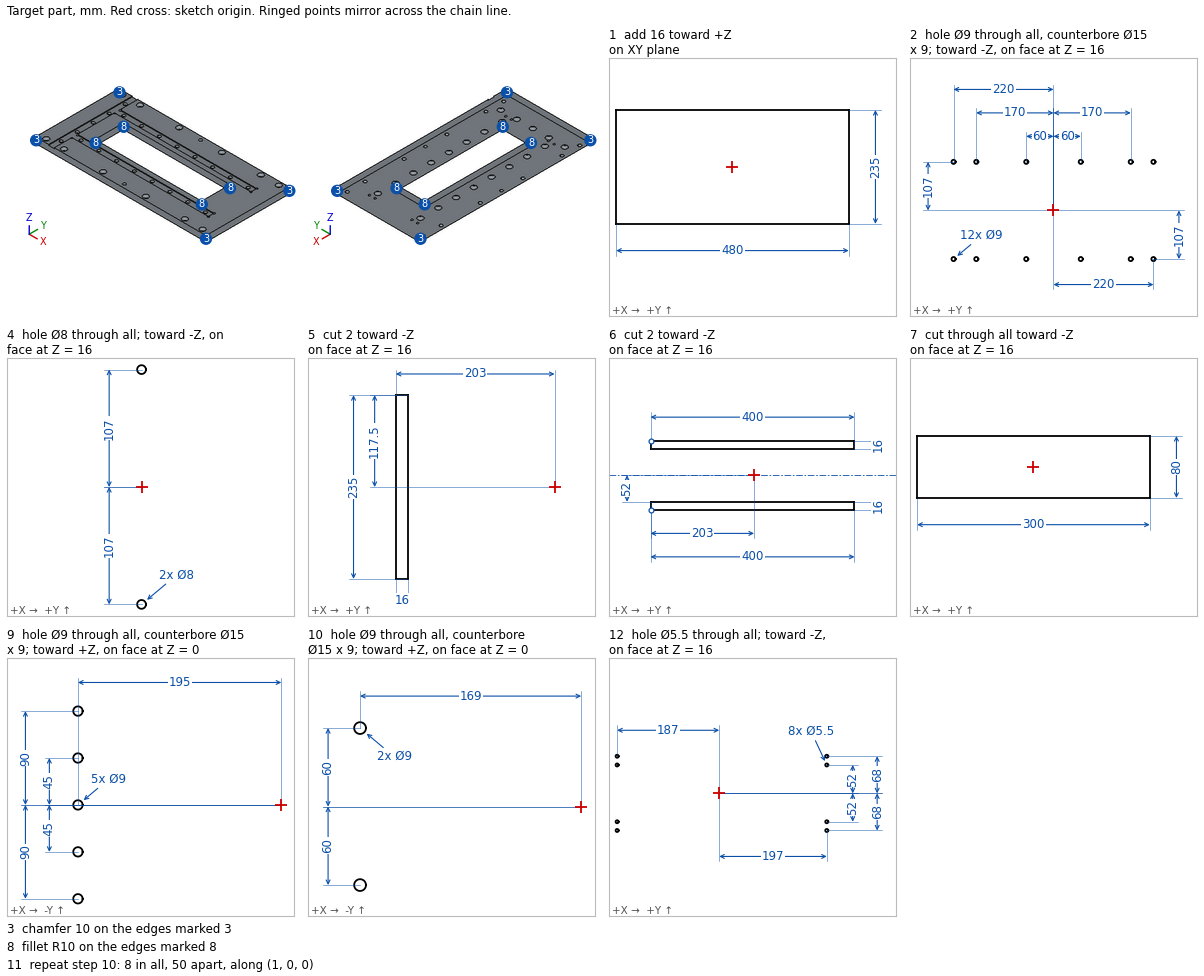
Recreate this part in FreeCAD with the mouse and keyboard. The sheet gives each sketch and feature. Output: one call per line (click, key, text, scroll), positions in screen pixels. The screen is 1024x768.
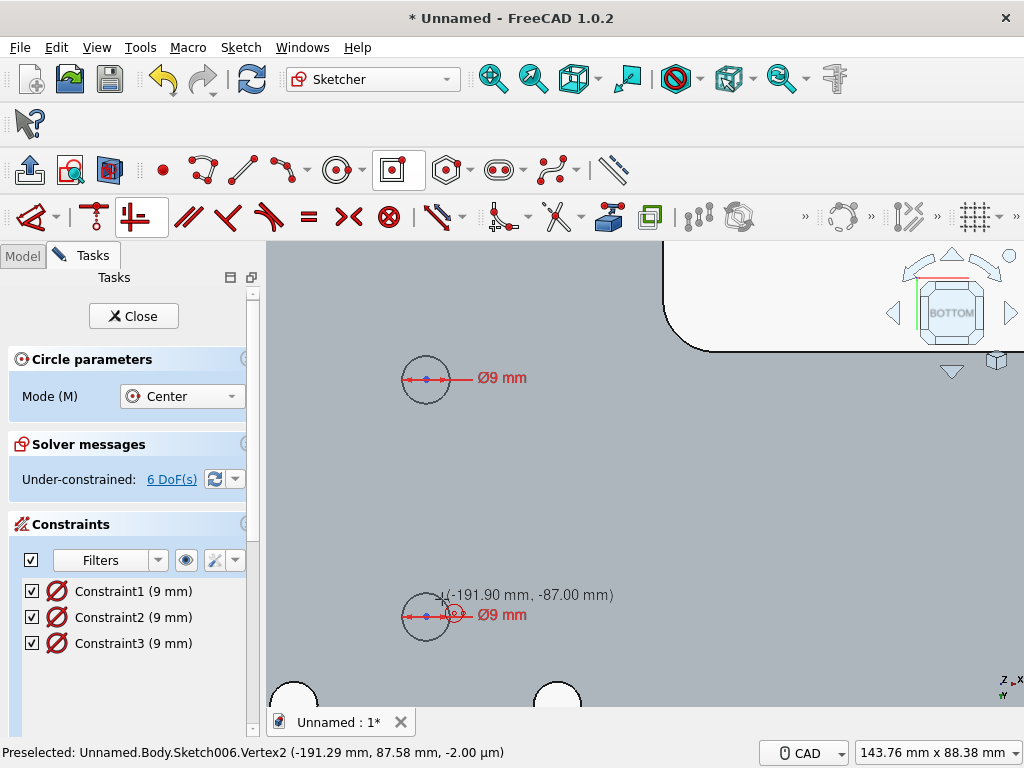
scroll(425, 617, down, 6)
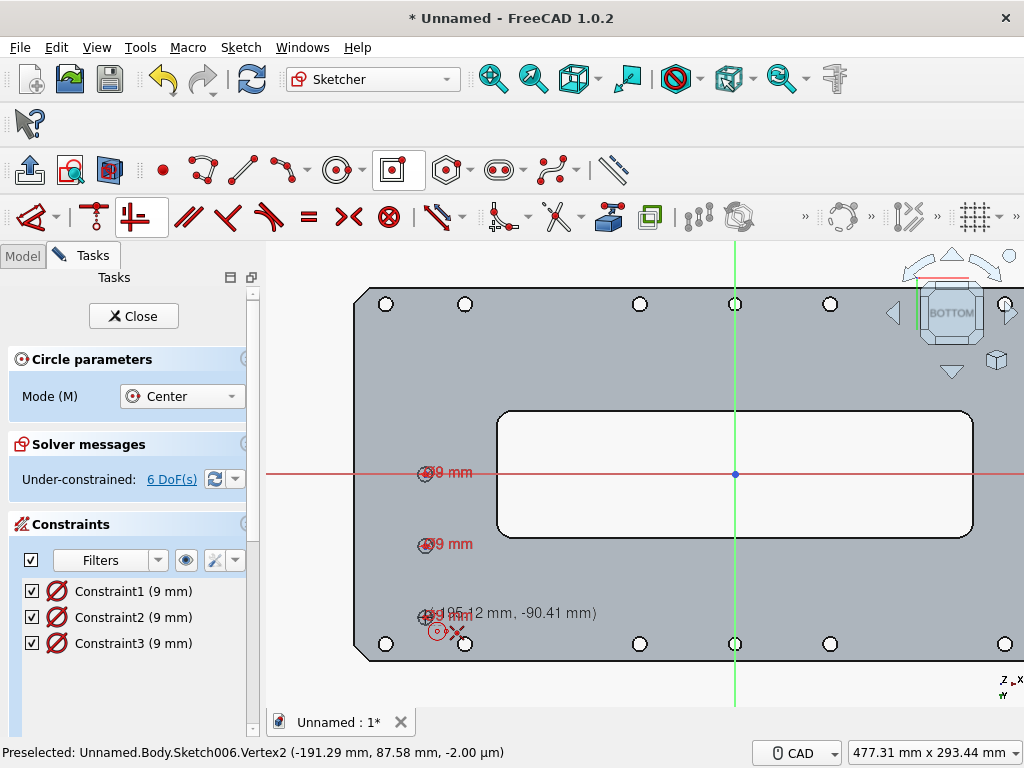
scroll(425, 331, up, 6)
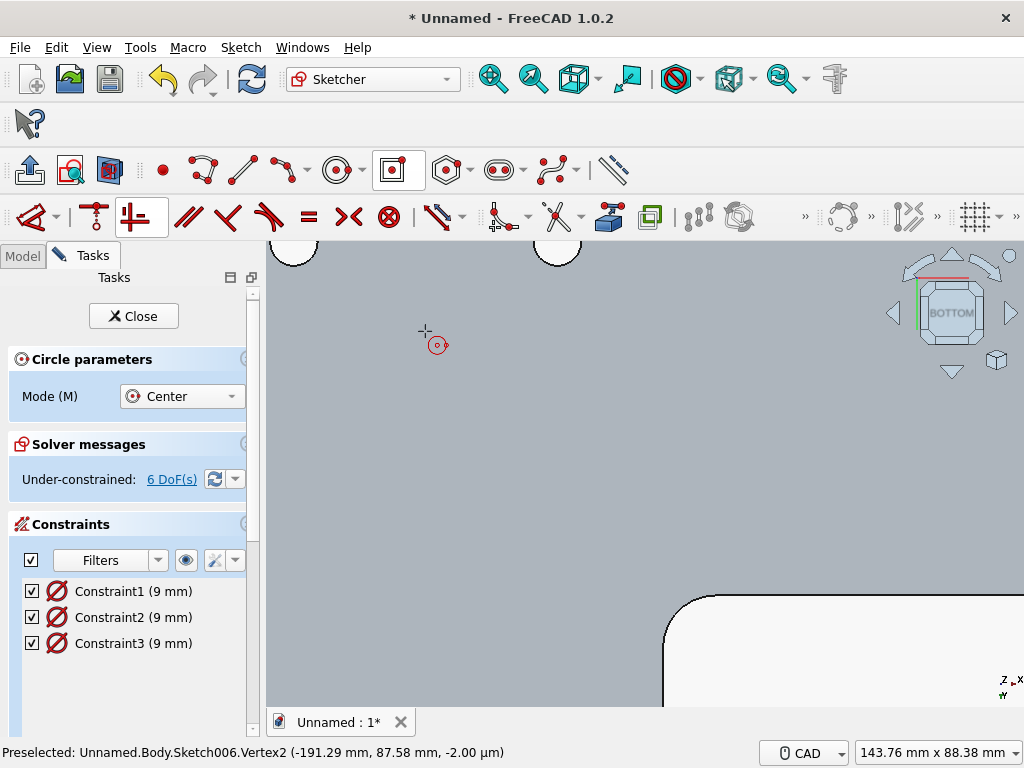
click(426, 332)
move(442, 315)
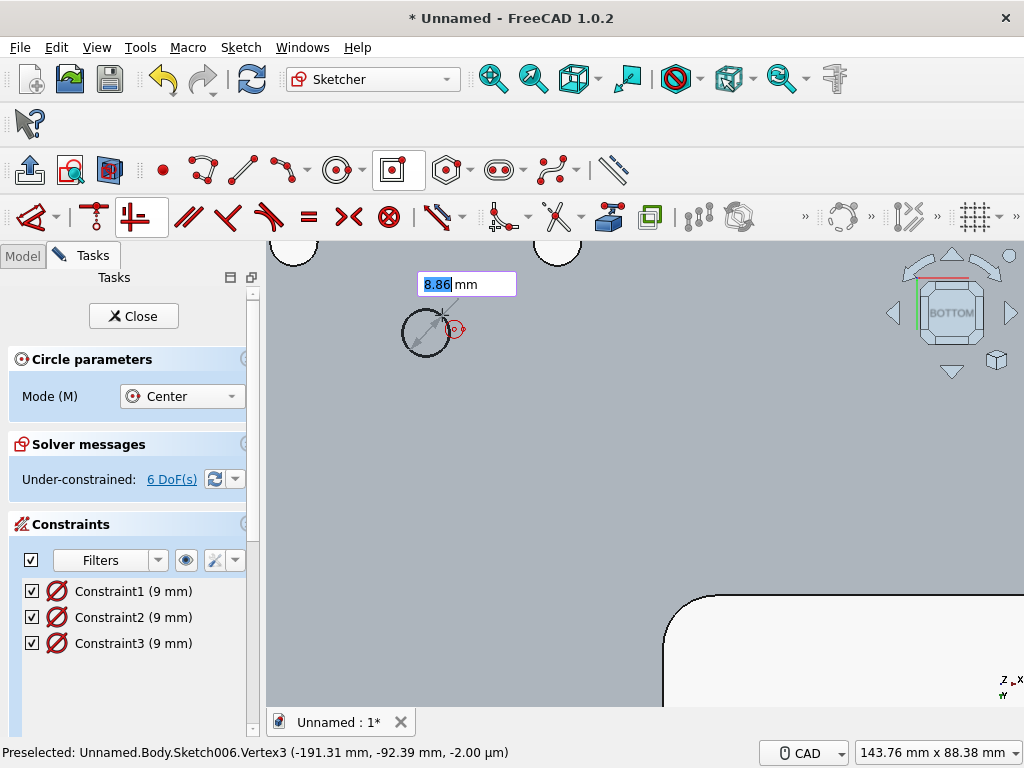
text(9)
key(Return)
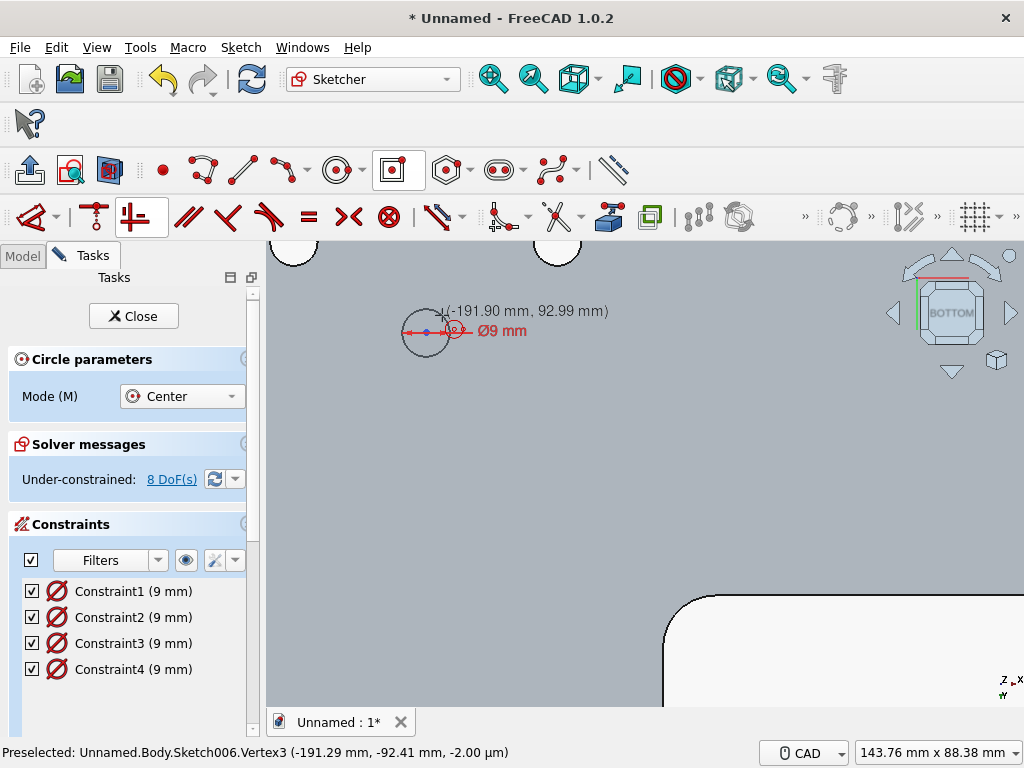
click(426, 569)
move(442, 552)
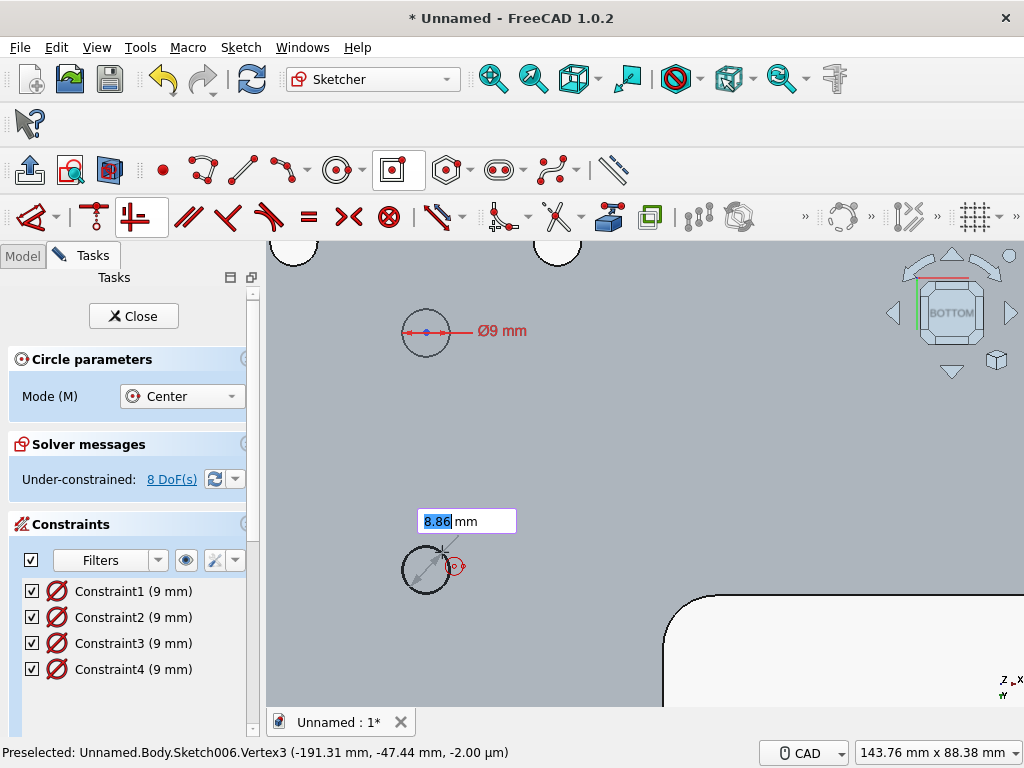
text(9)
key(Return)
key(Escape)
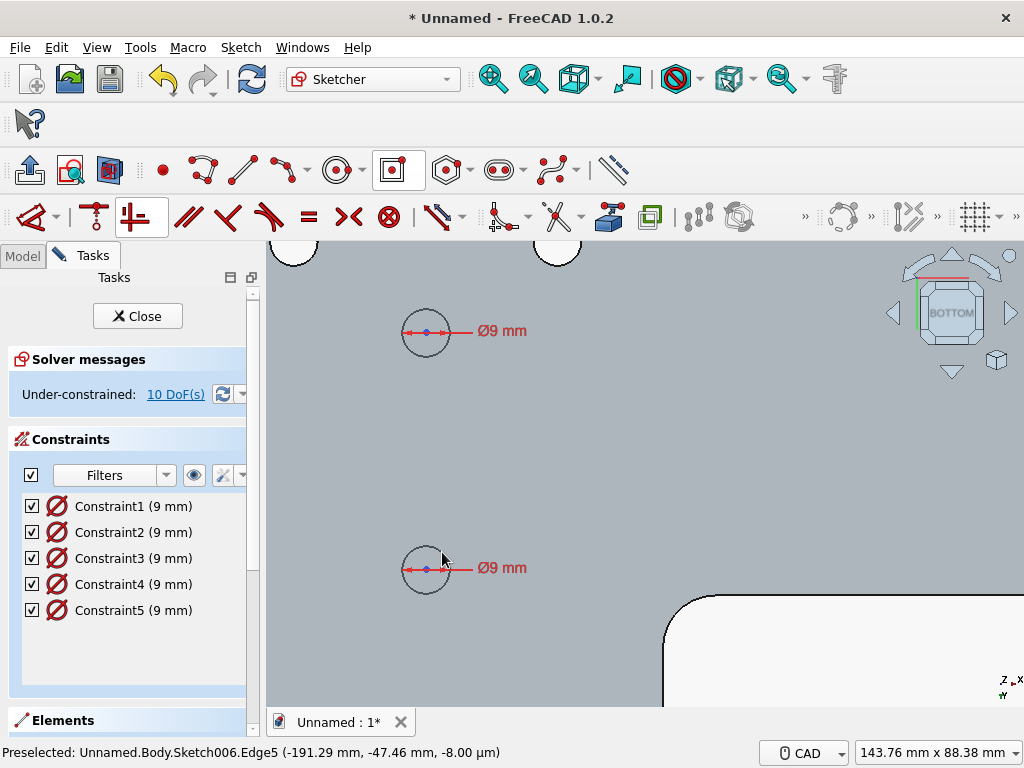
scroll(425, 331, down, 6)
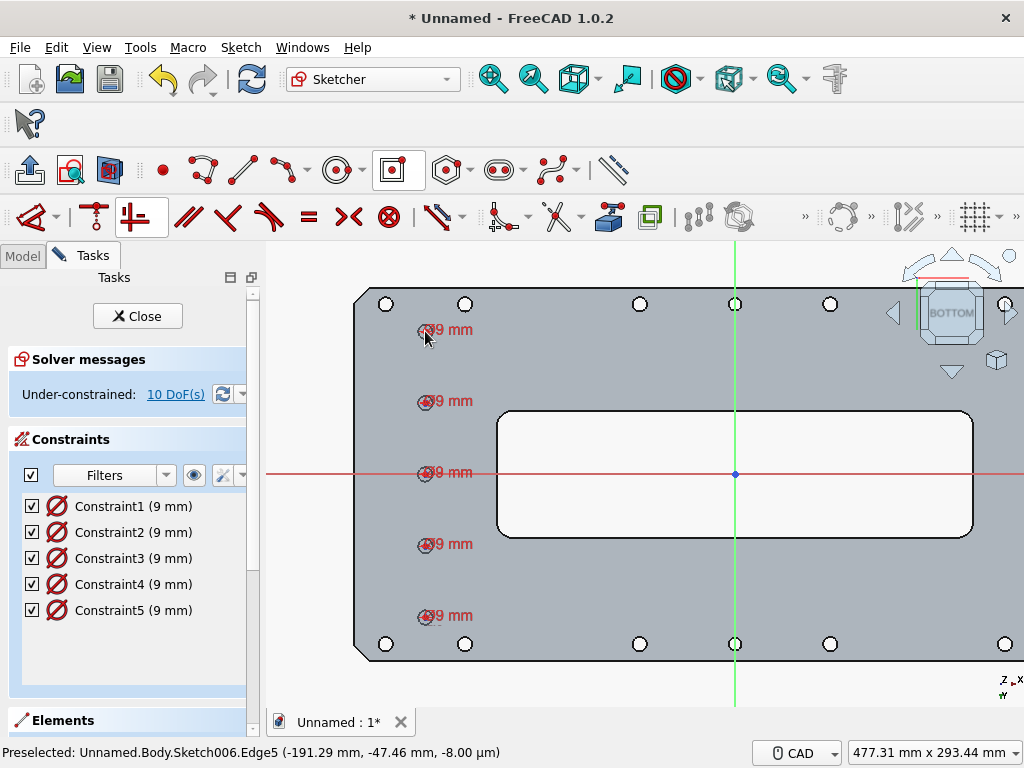
click(425, 474)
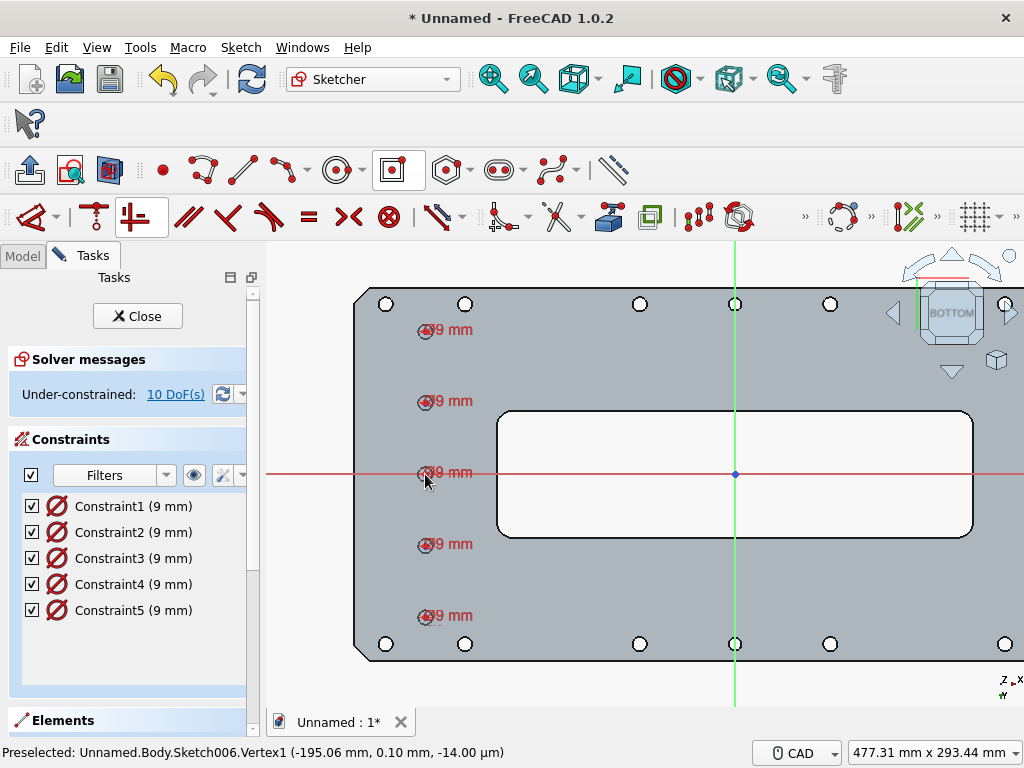
click(334, 474)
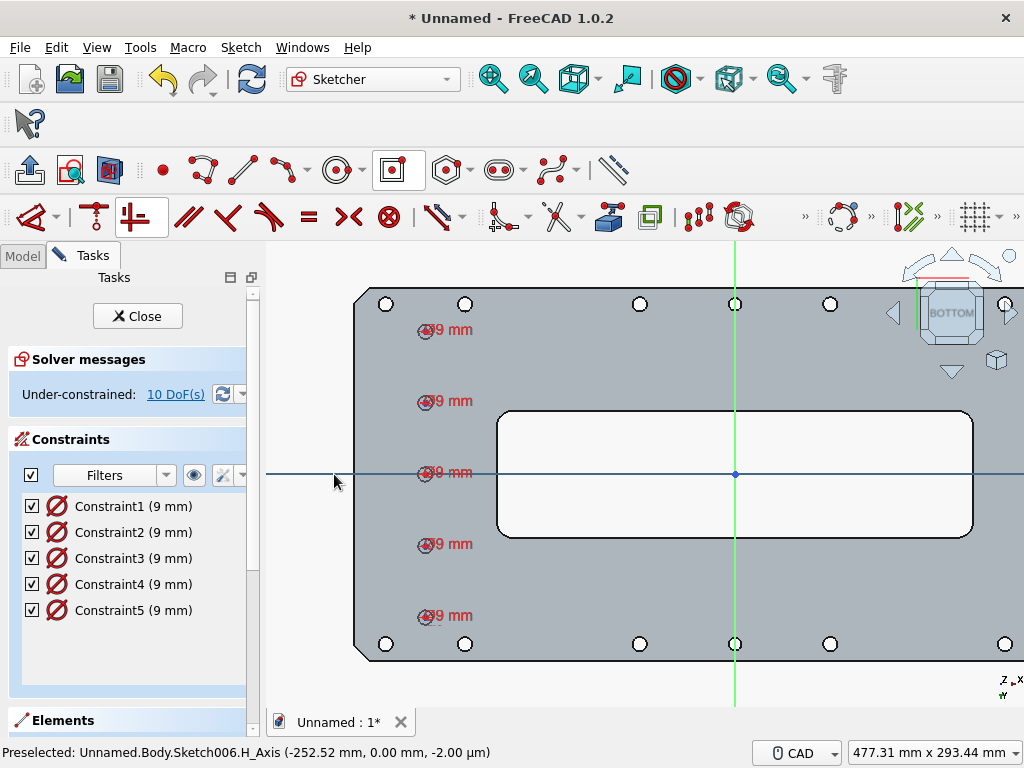
click(94, 218)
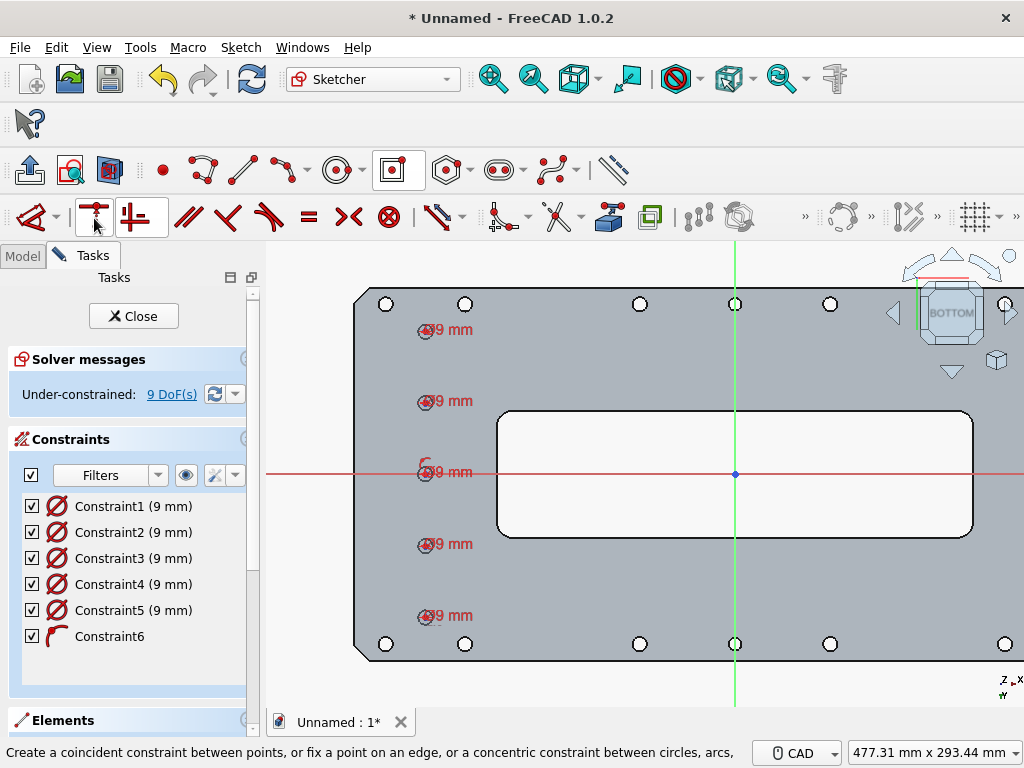
click(425, 474)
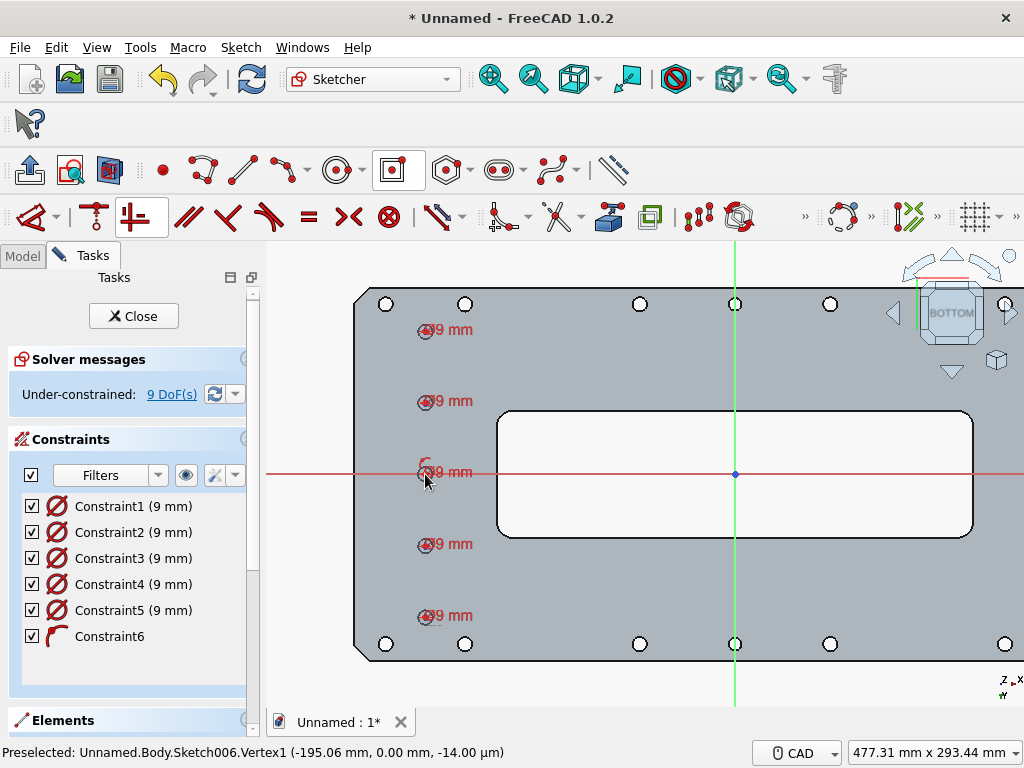
click(425, 546)